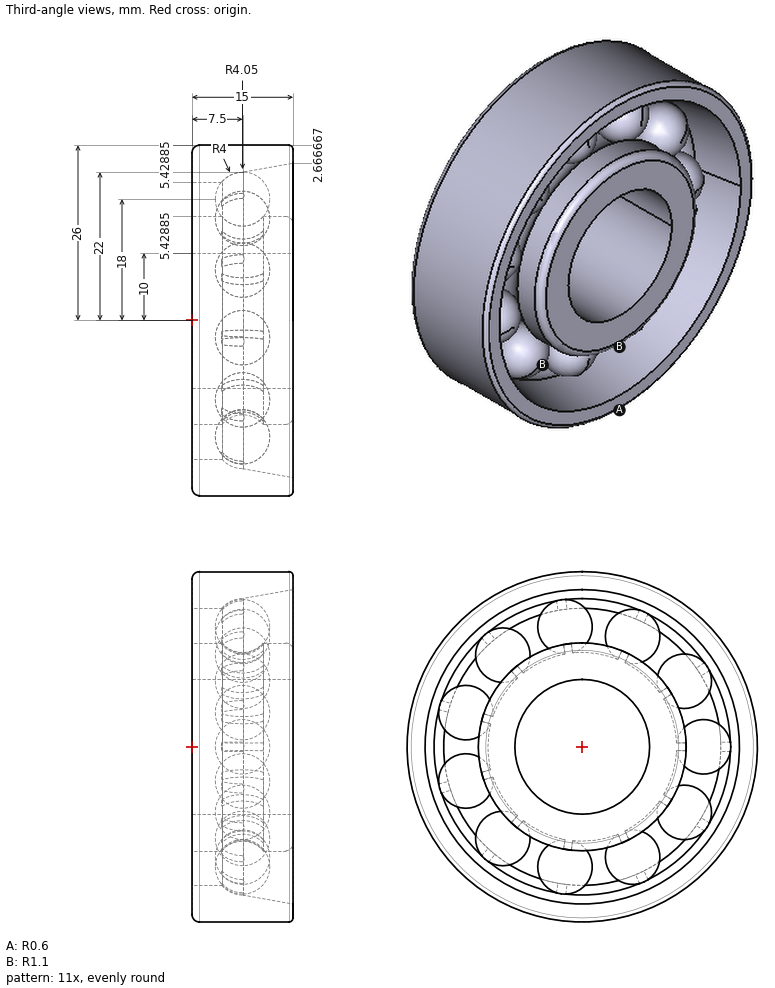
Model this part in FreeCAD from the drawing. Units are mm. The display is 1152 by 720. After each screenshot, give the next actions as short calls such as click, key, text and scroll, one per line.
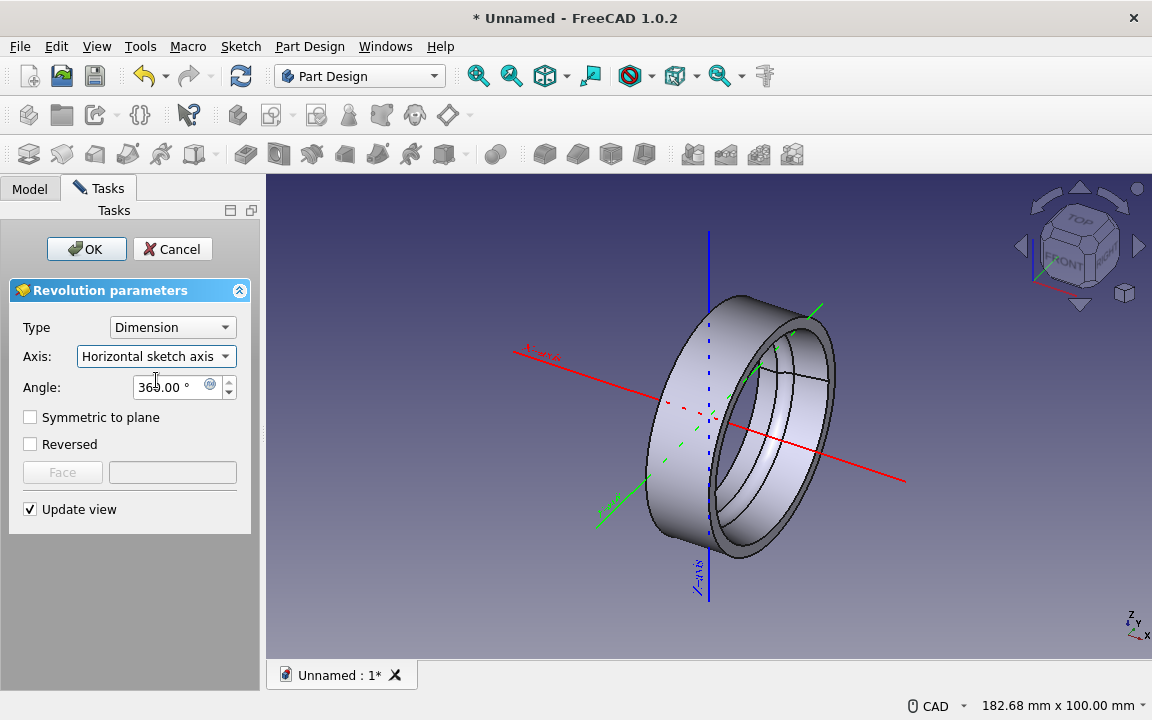
click(87, 249)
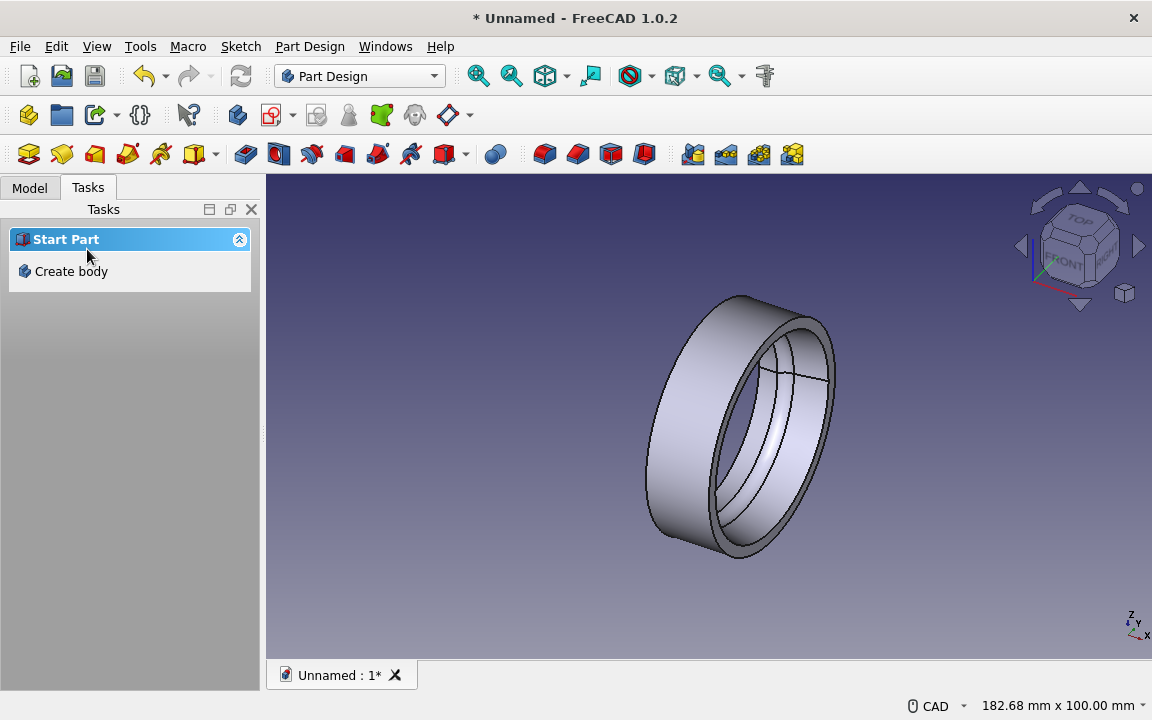
click(270, 116)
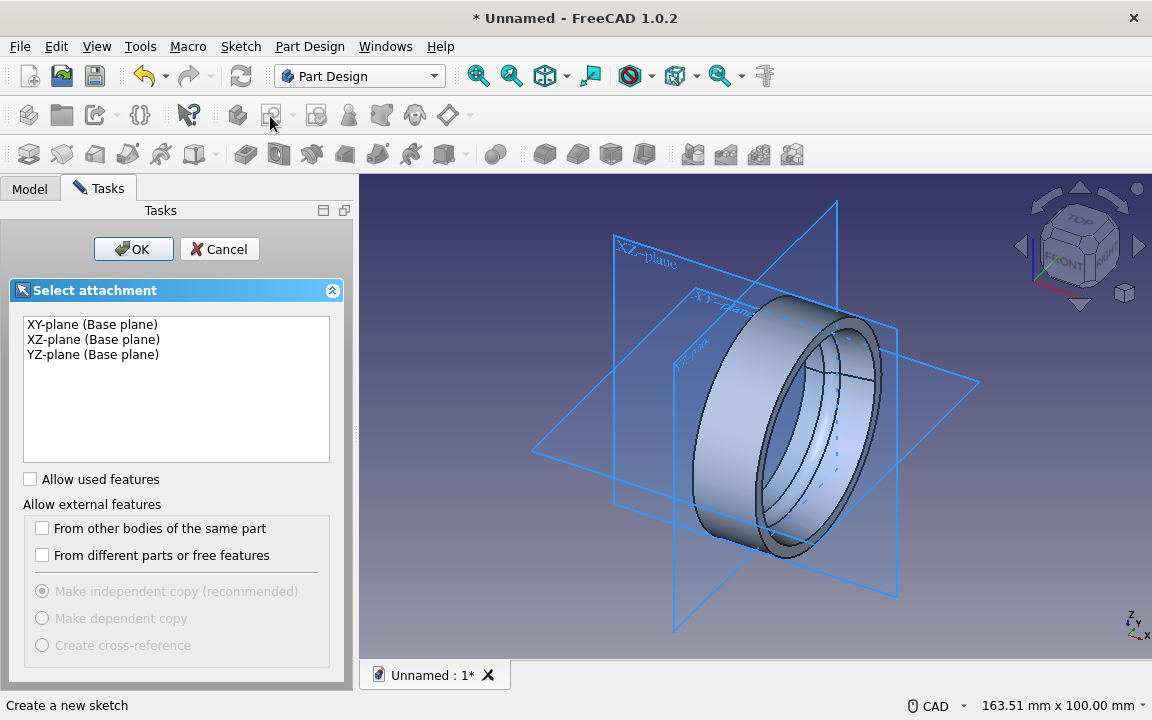
click(84, 324)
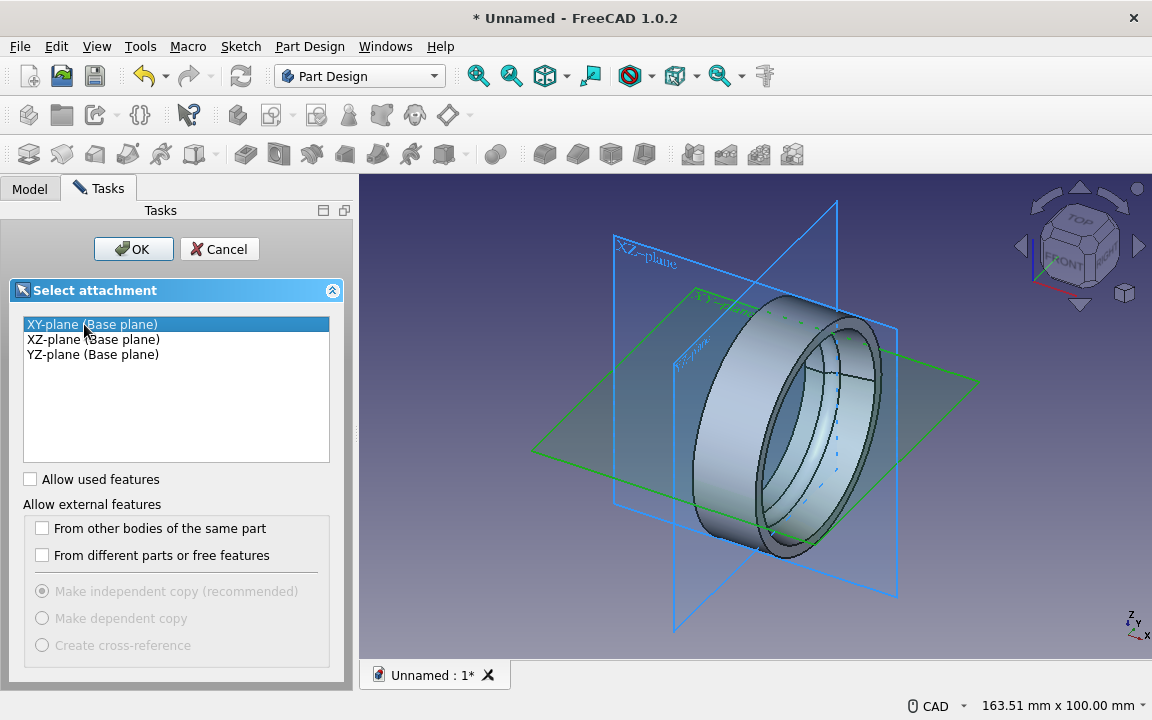
click(134, 249)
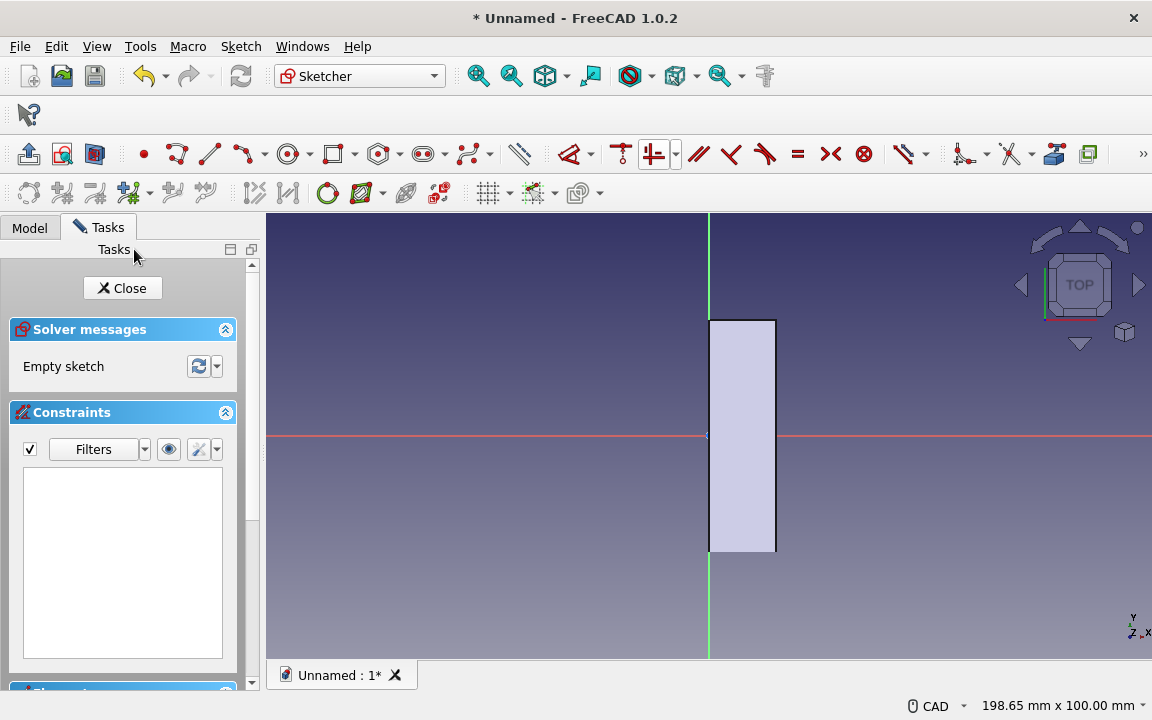
click(95, 154)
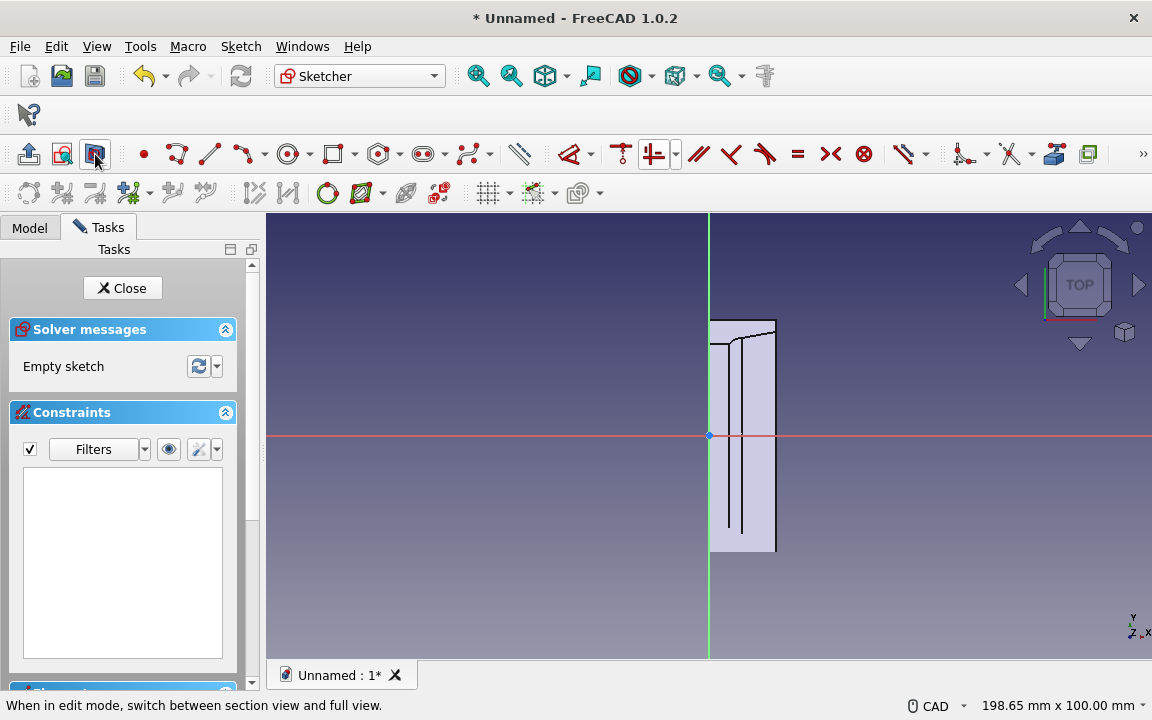
scroll(801, 358, up, 5)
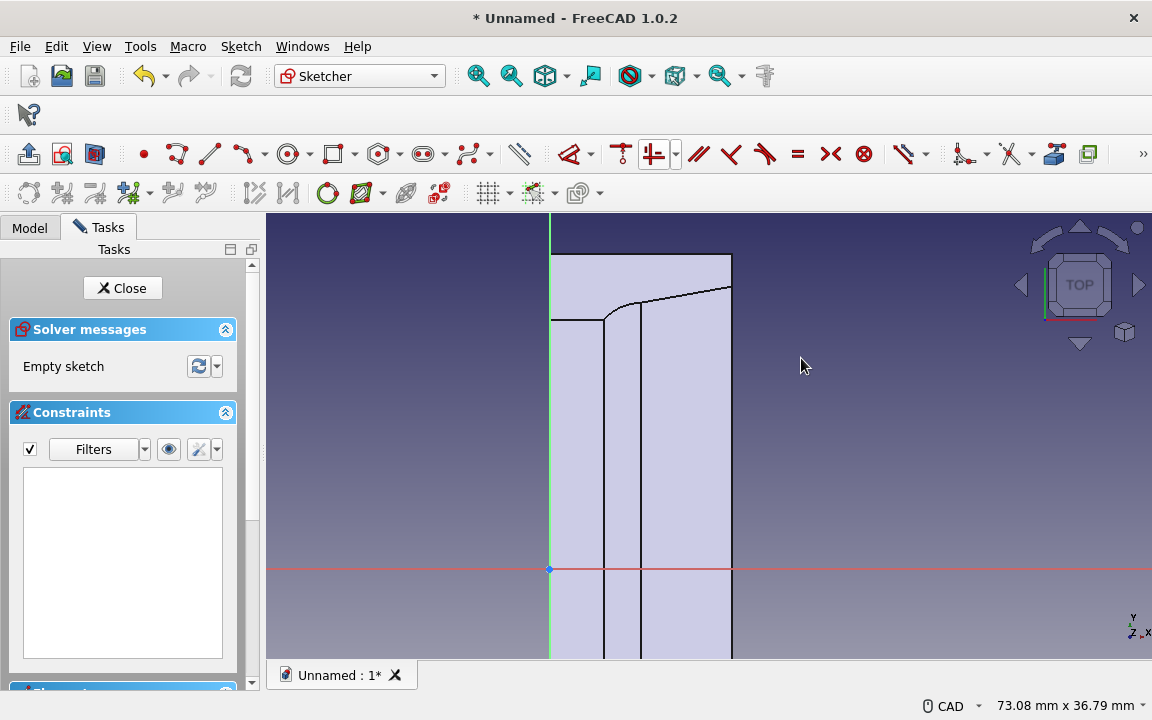
click(210, 154)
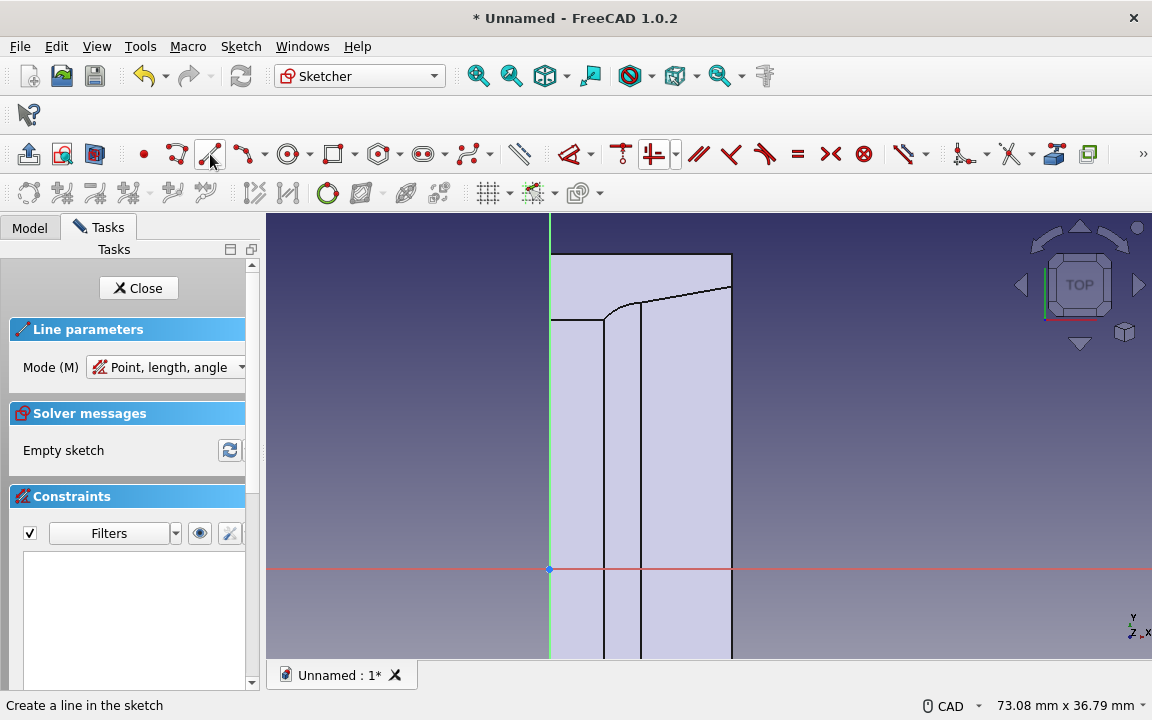
click(592, 351)
click(690, 351)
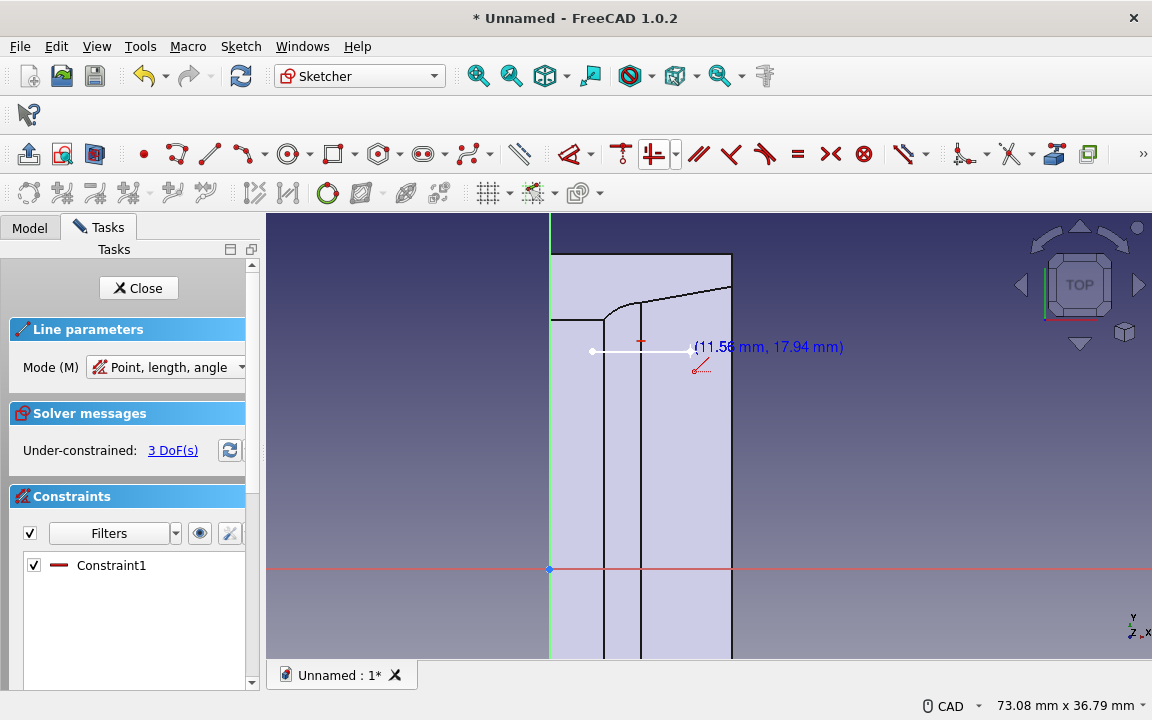
click(242, 154)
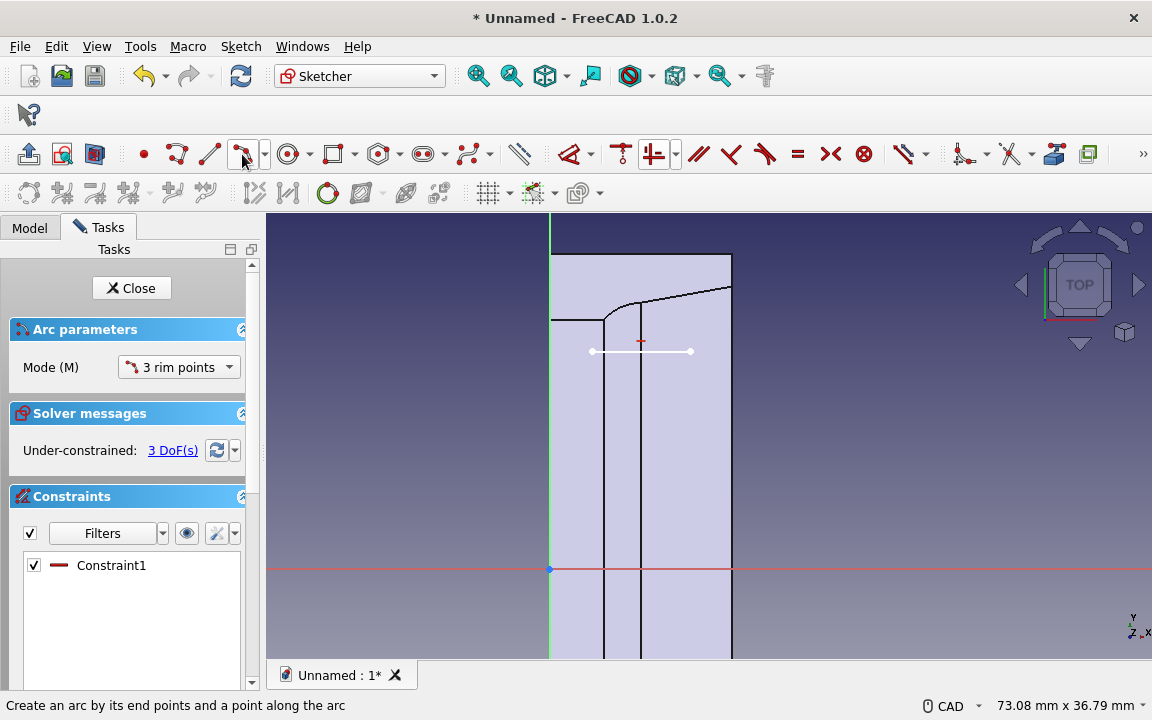
click(690, 352)
click(592, 352)
click(641, 302)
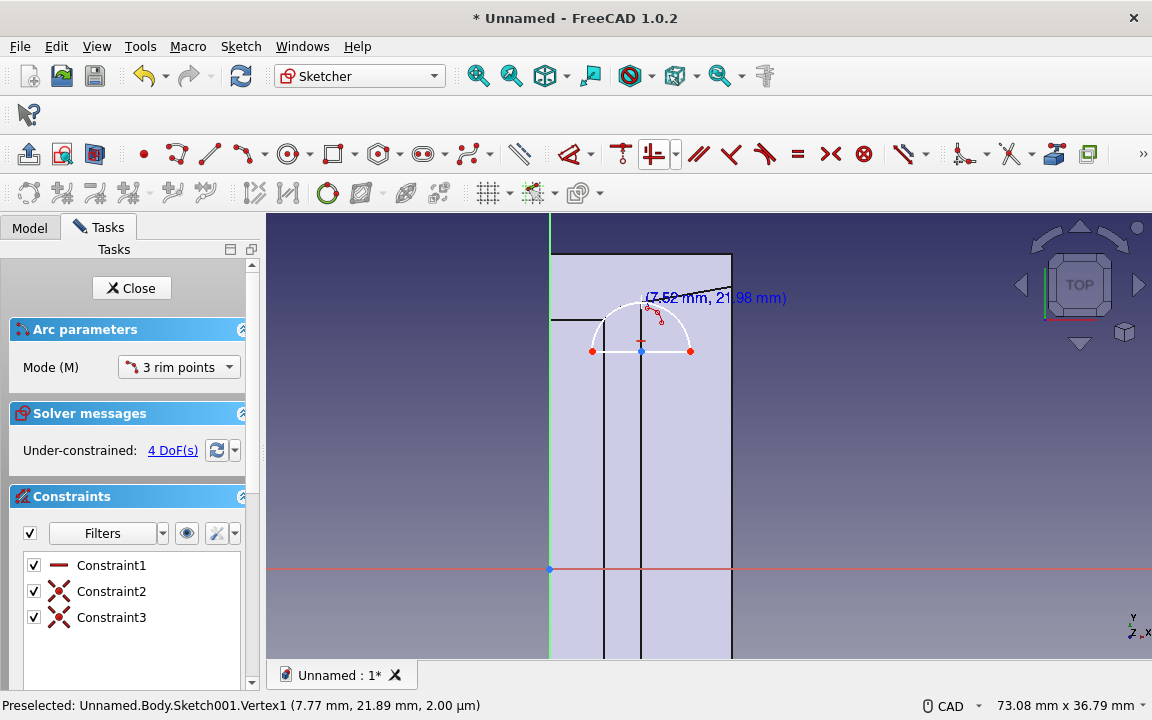
click(210, 154)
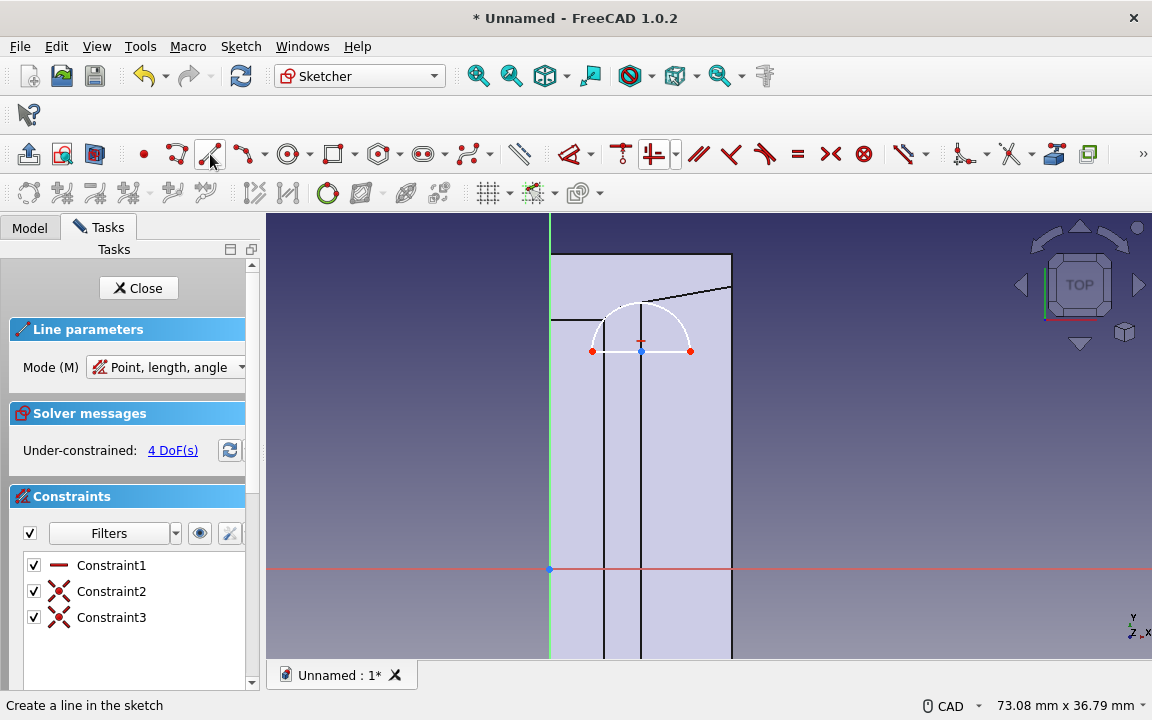
scroll(700, 351, up, 3)